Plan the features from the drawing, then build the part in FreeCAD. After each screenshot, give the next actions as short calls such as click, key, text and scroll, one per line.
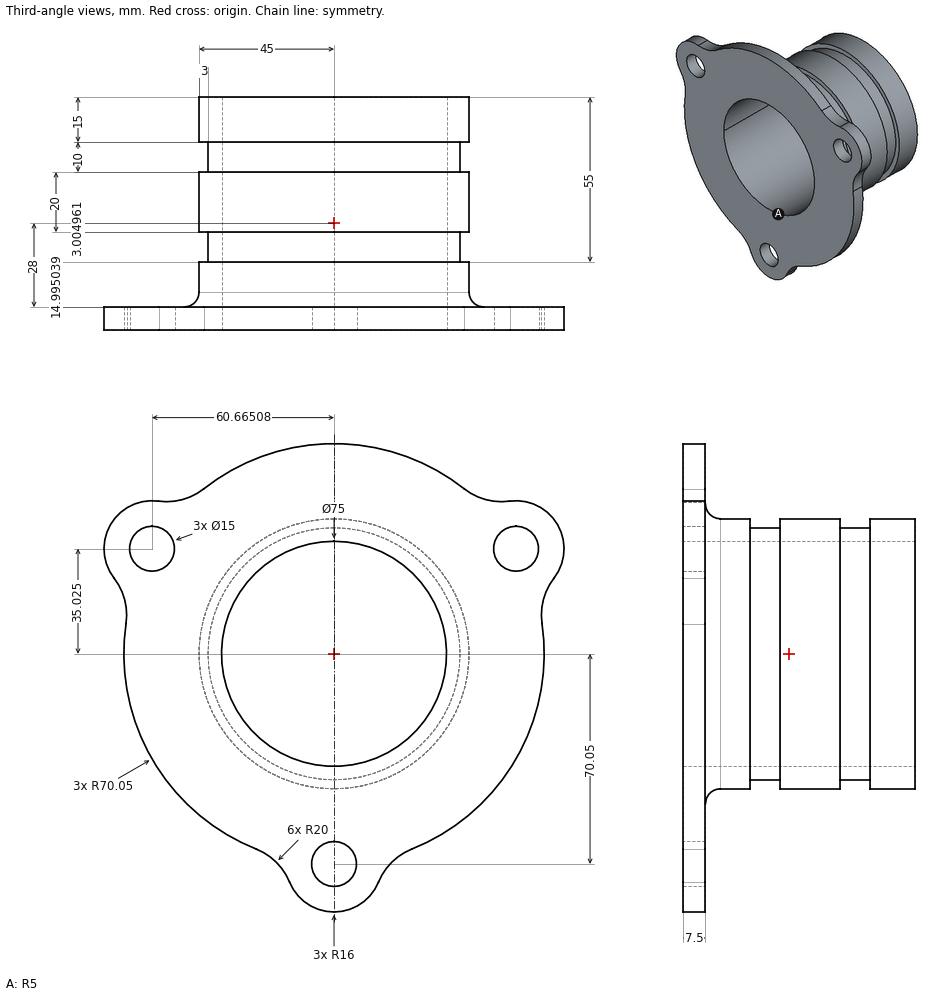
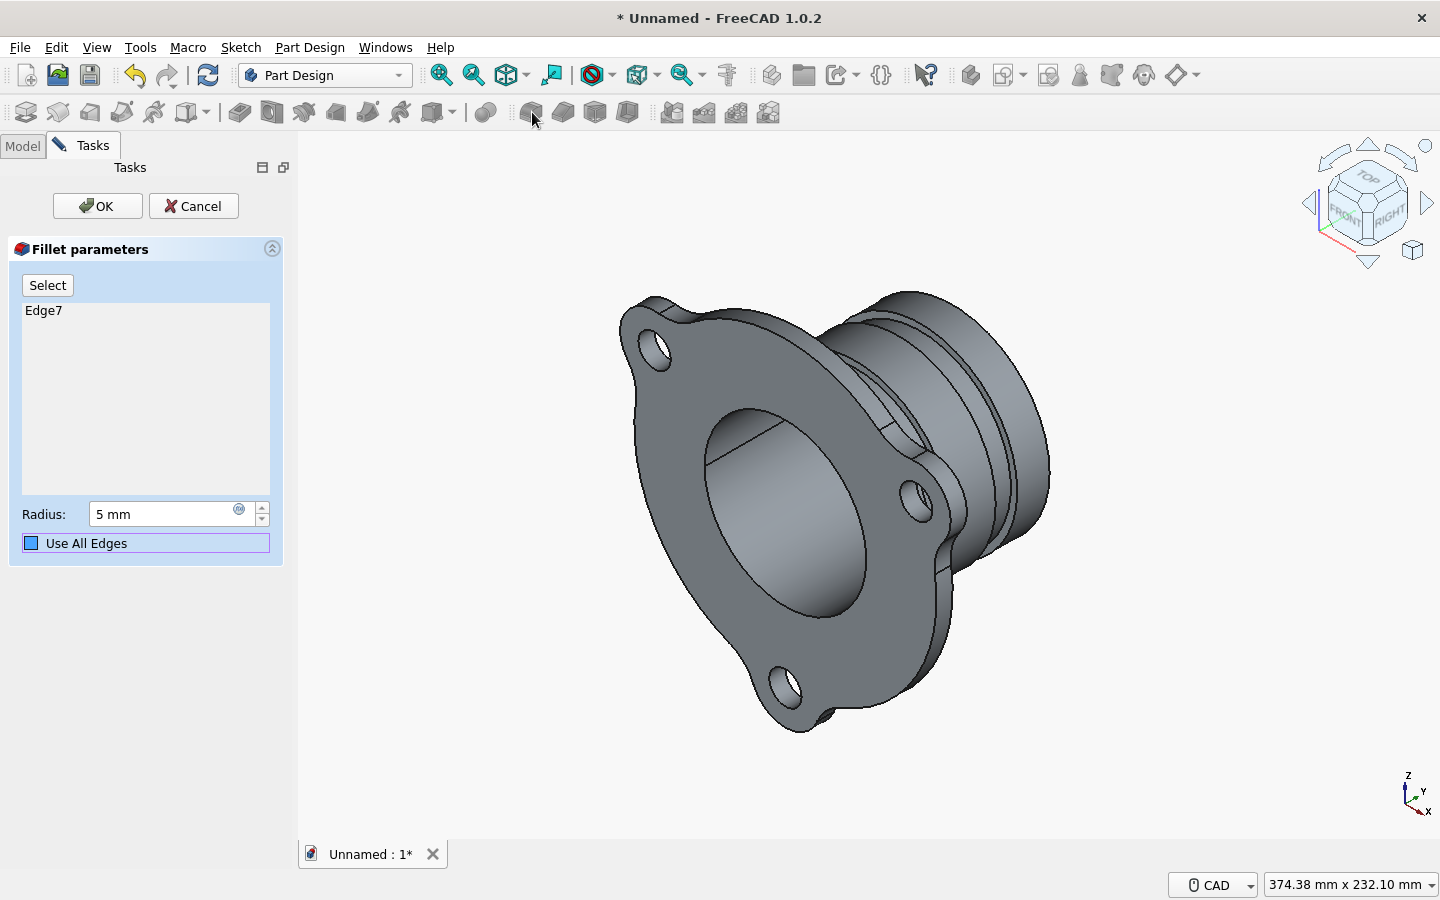
click(98, 206)